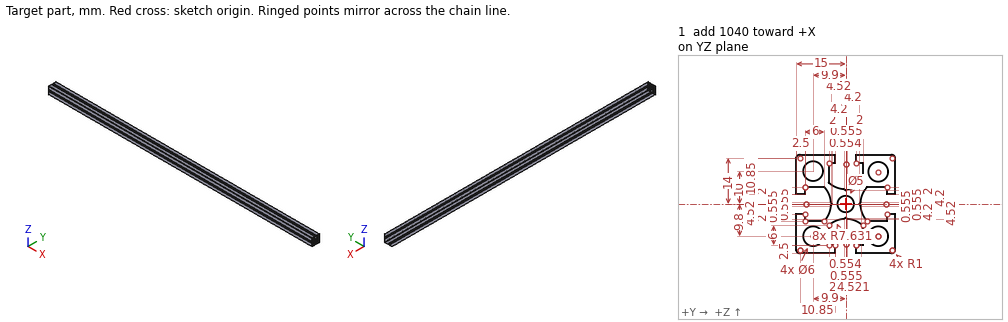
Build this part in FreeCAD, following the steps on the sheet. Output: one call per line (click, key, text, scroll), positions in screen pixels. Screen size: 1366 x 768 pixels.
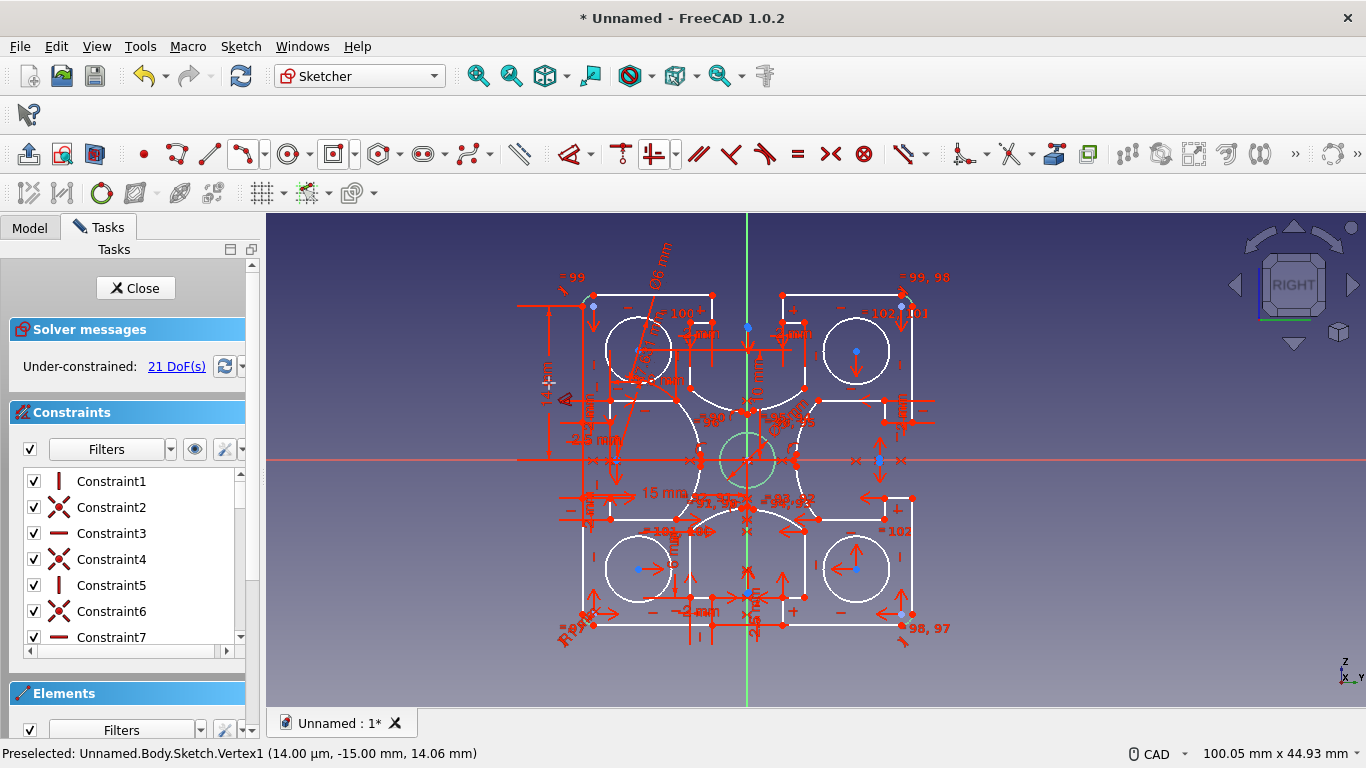
click(639, 350)
click(731, 292)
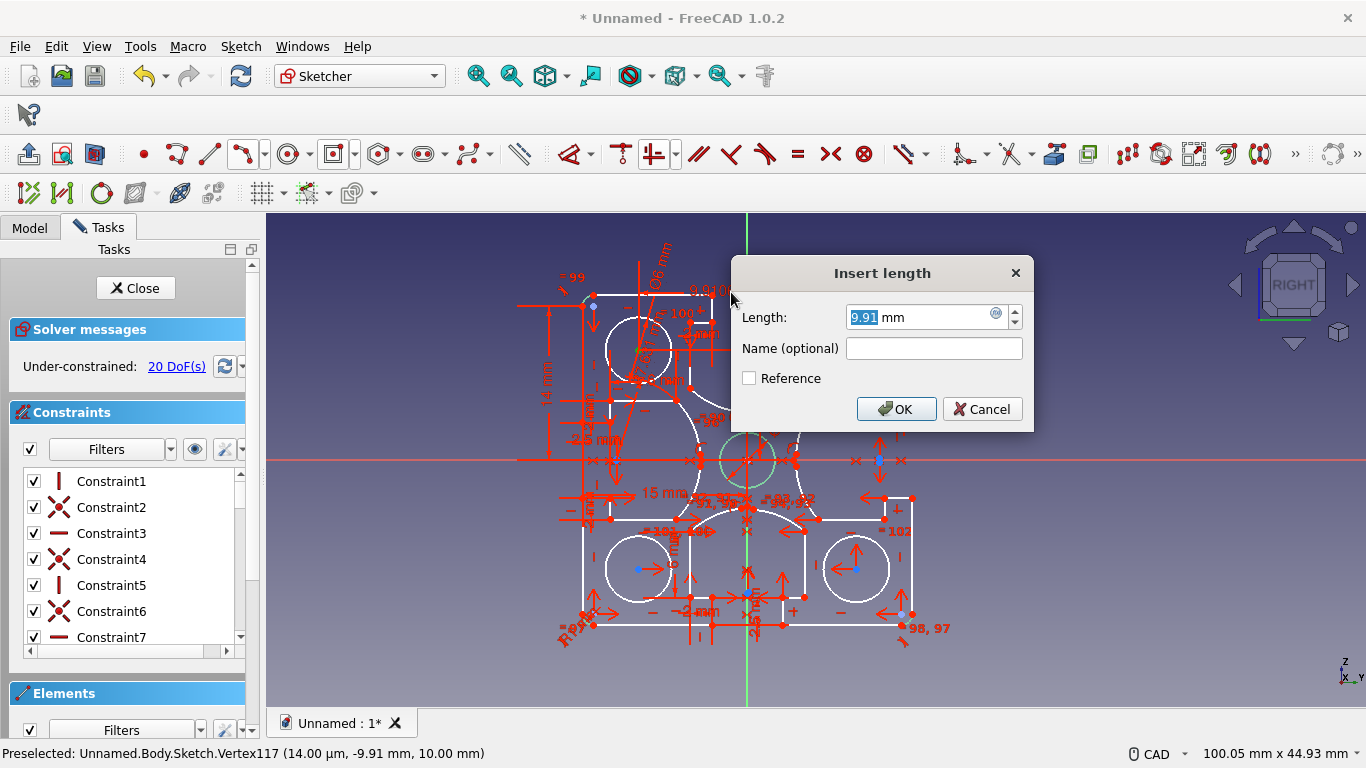
text(9.9)
key(Return)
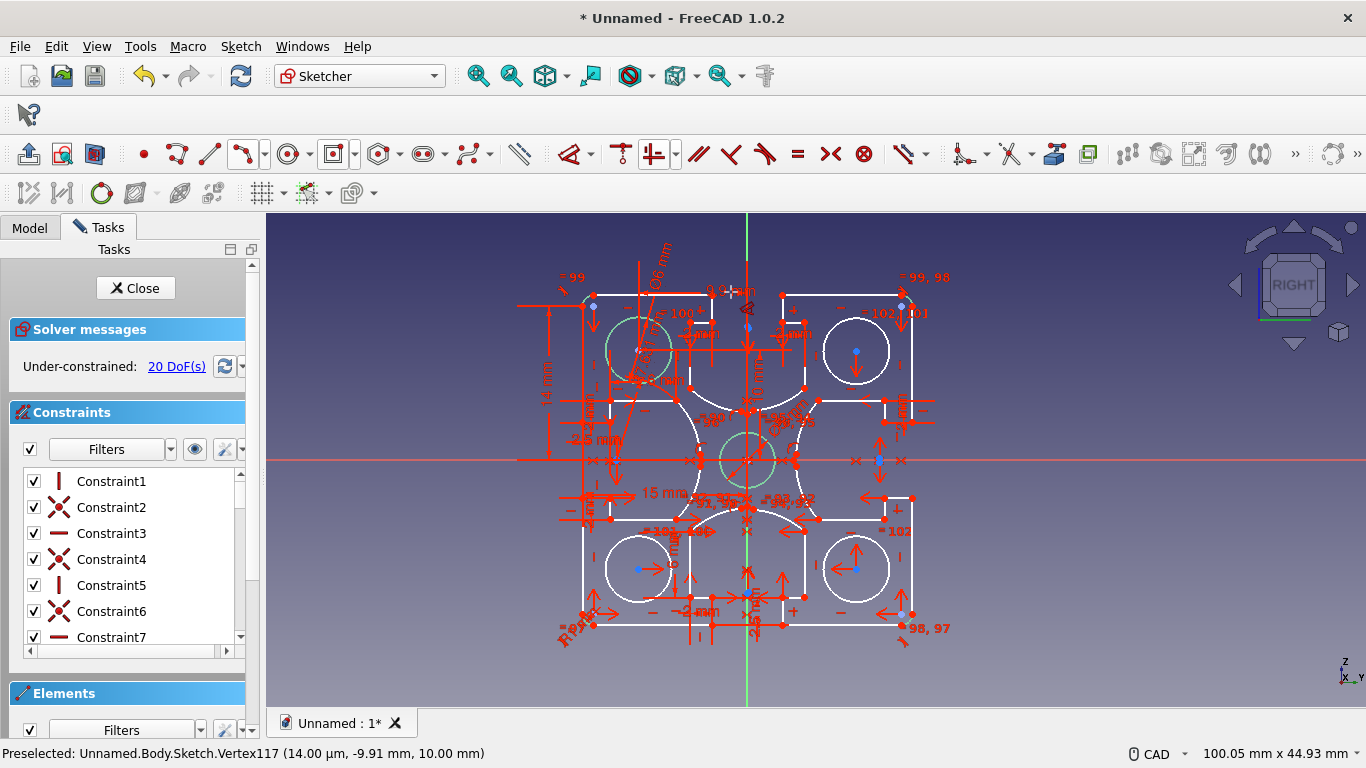
click(639, 569)
click(668, 426)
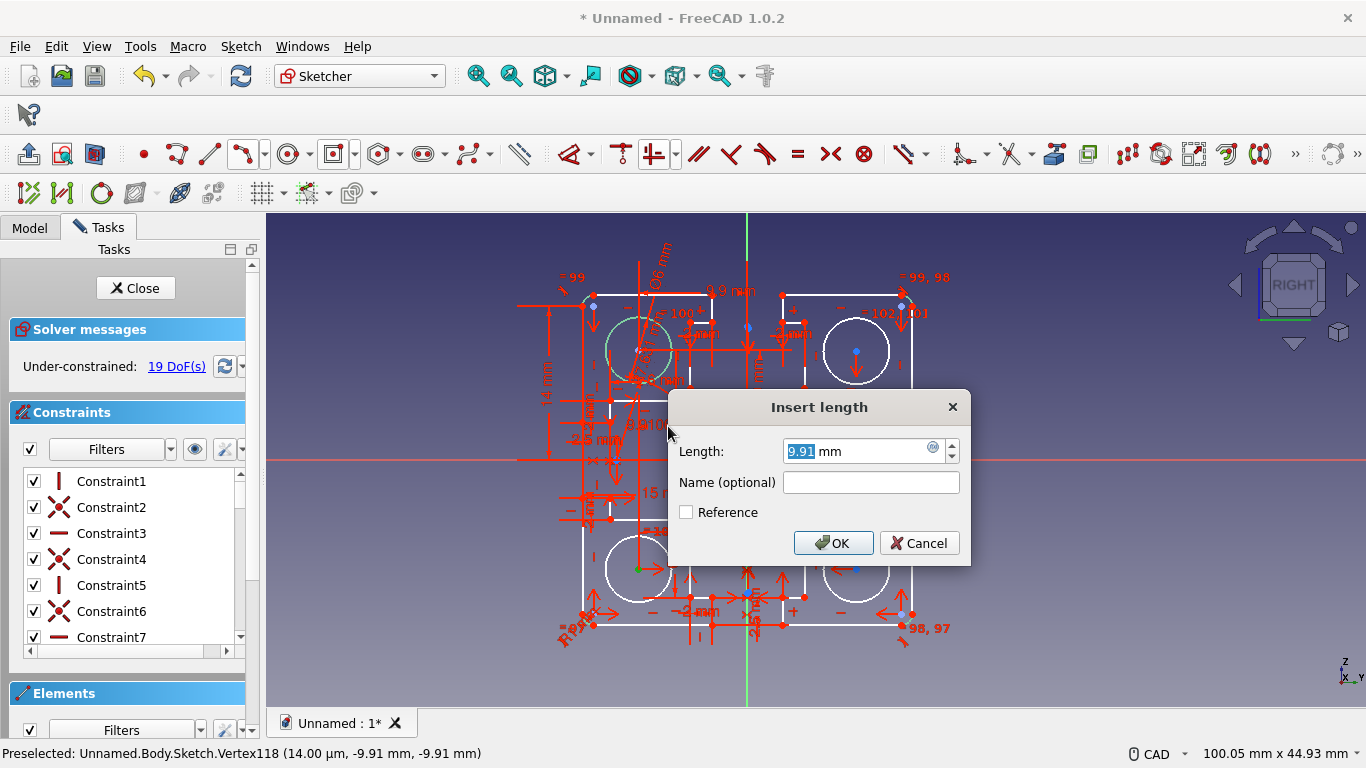
text(9.9)
key(Return)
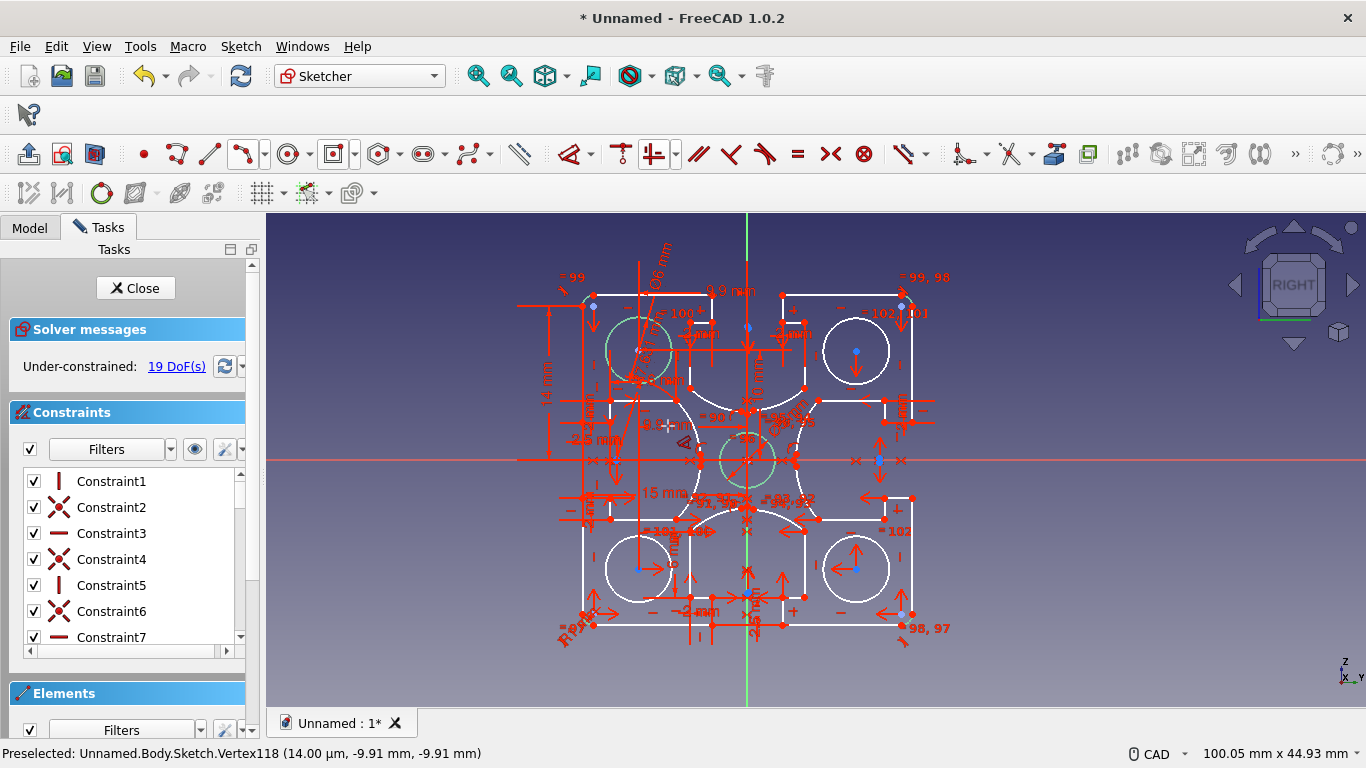
click(639, 569)
click(781, 490)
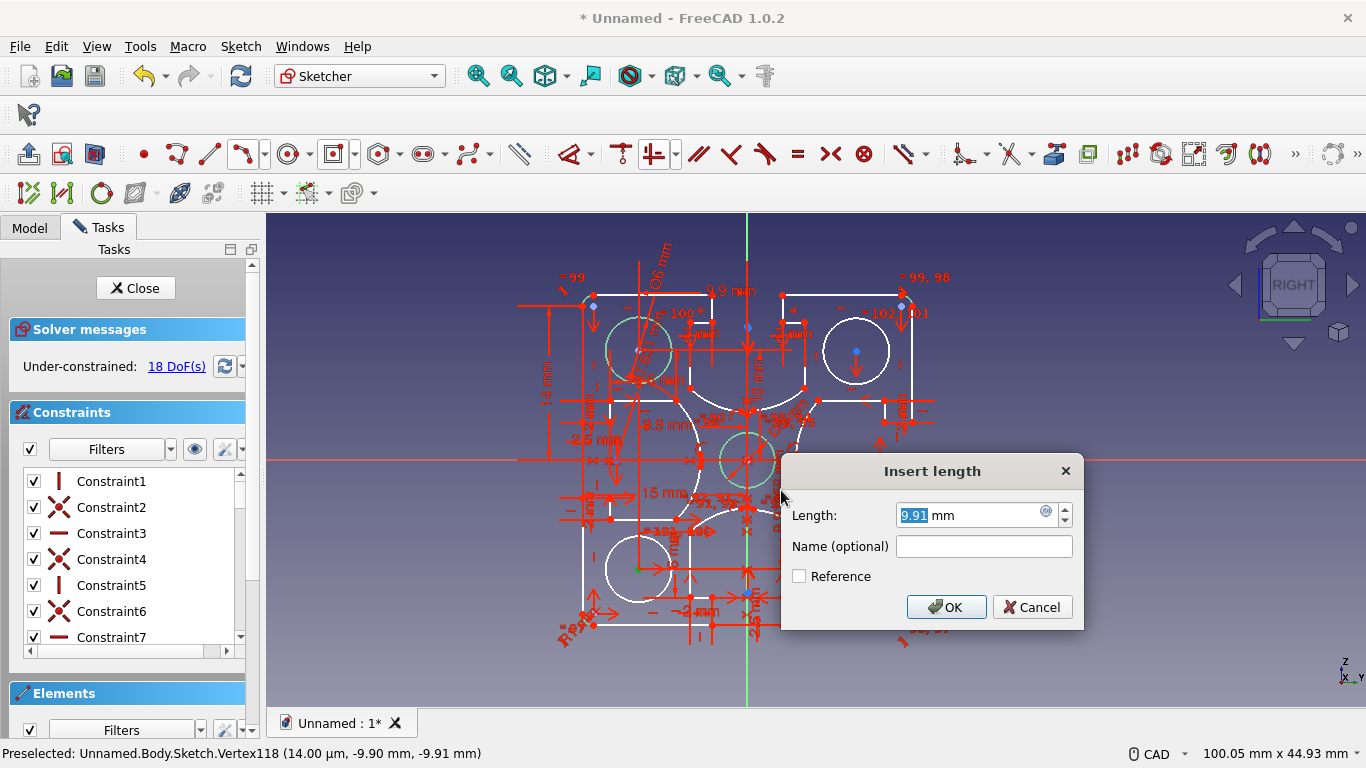
text(9.8)
key(Return)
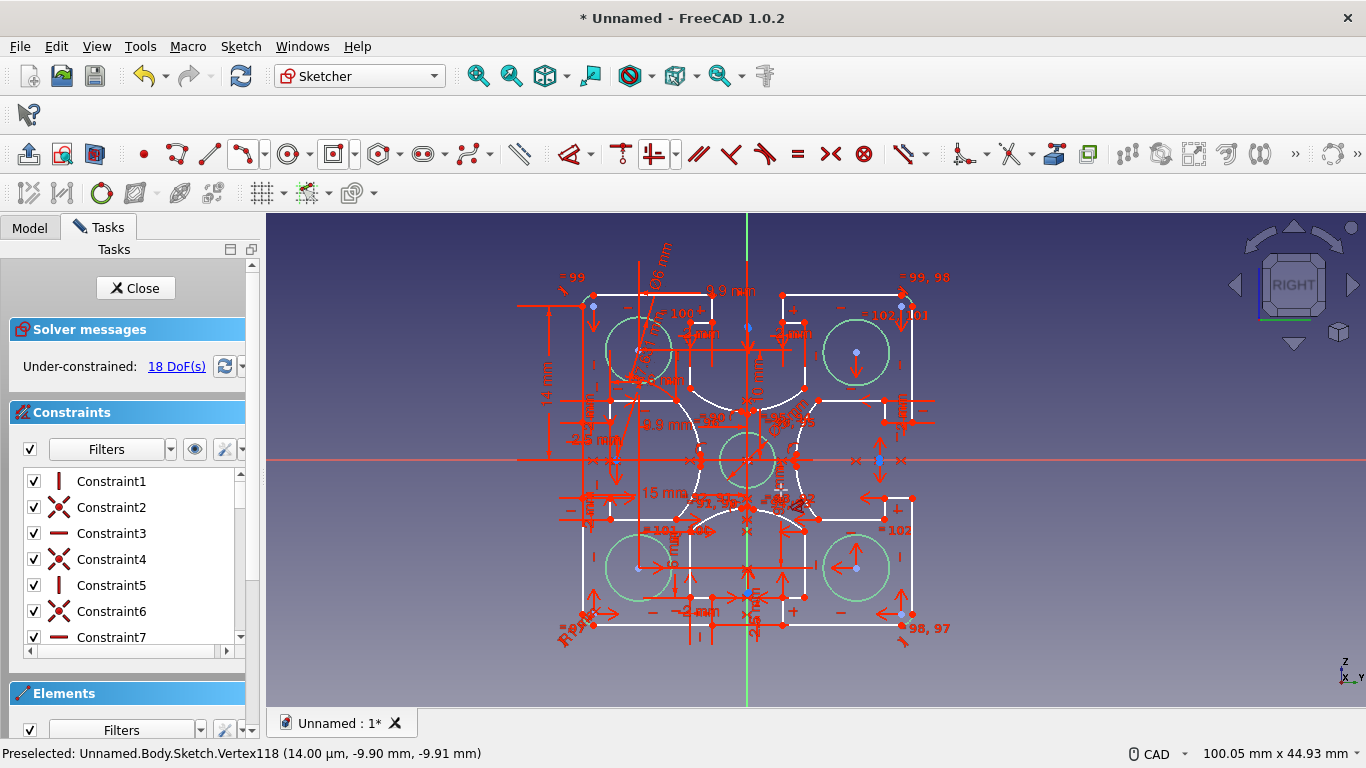
scroll(701, 460, up, 4)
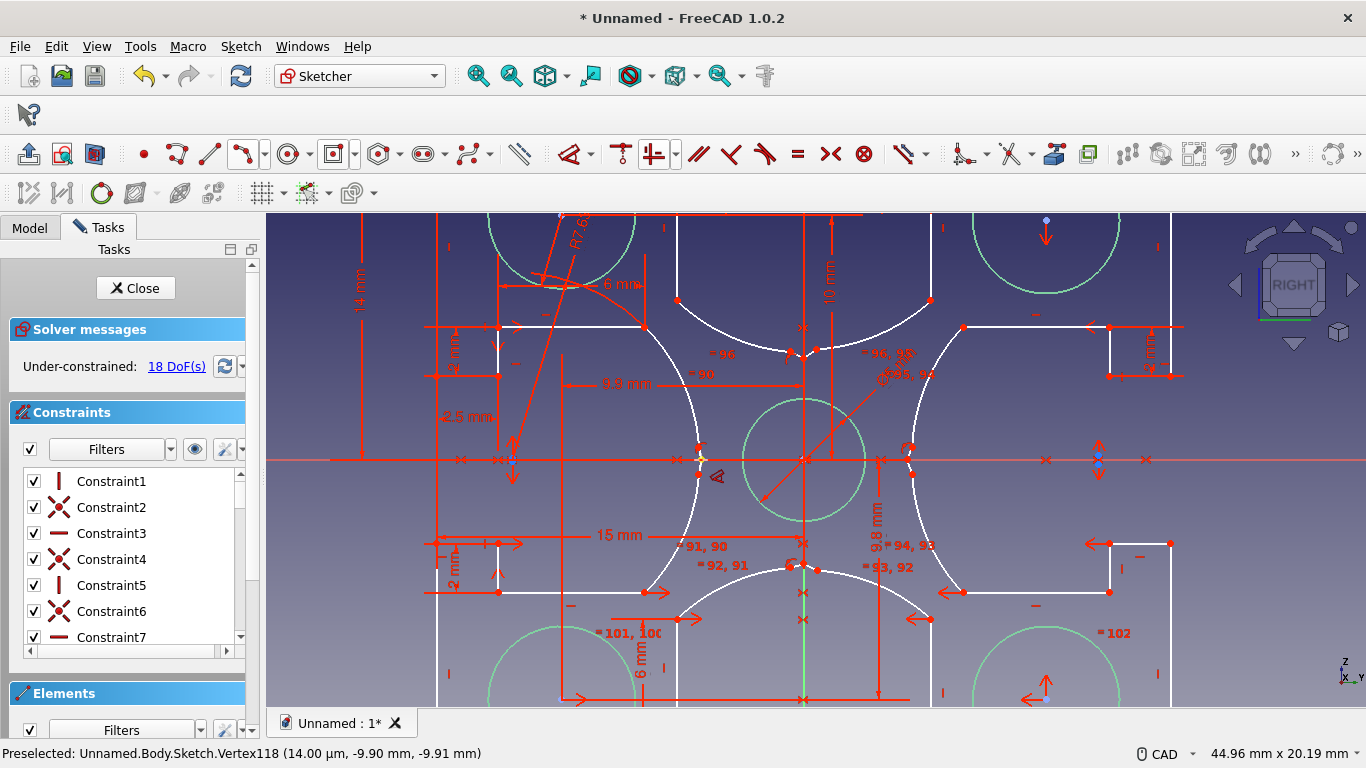
click(701, 460)
click(729, 494)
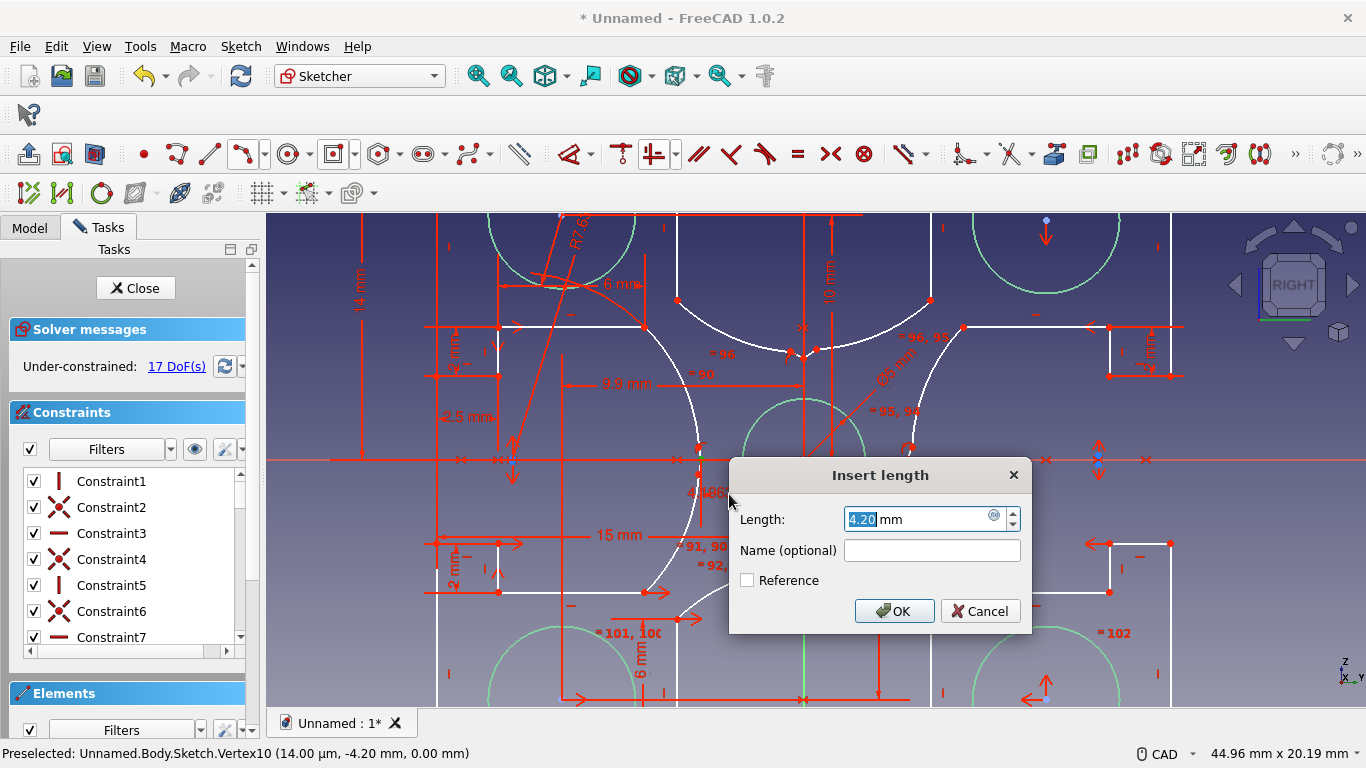
text(4.2)
key(Return)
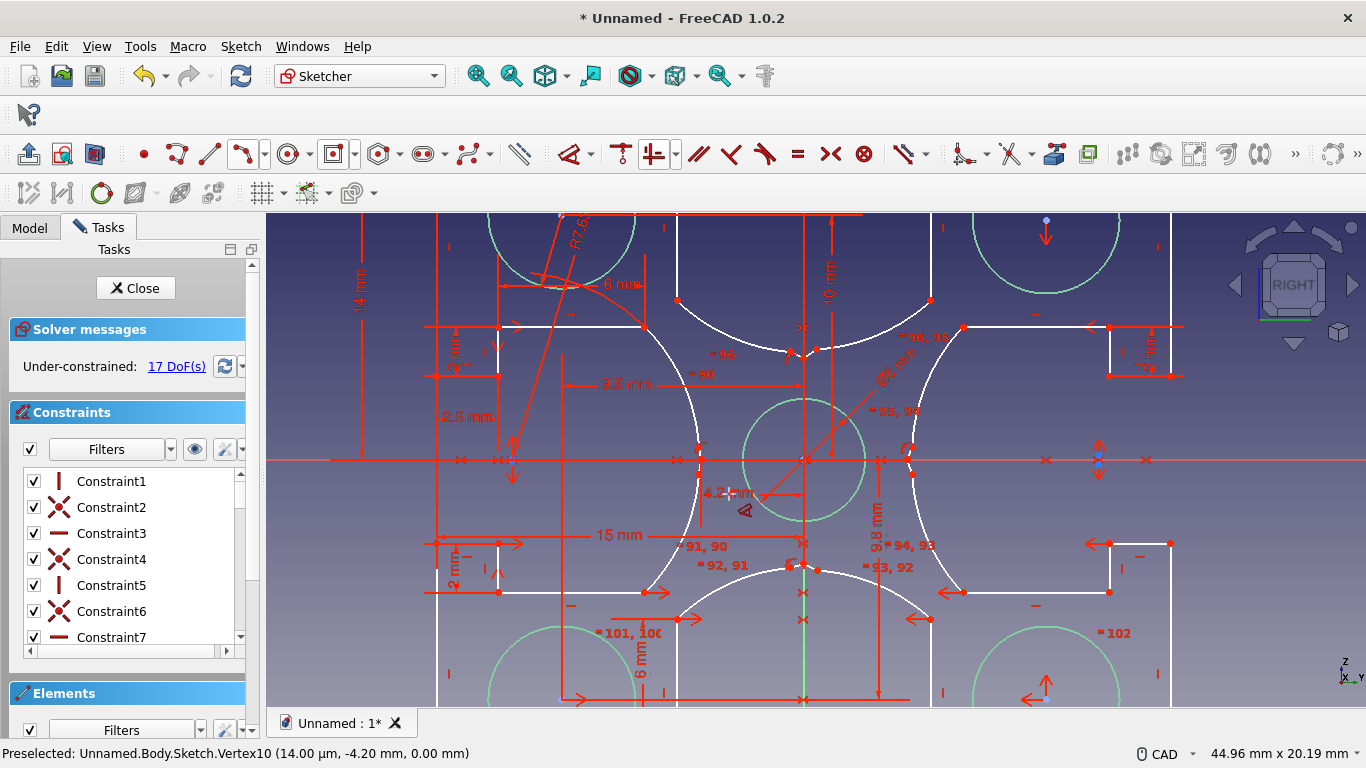
click(804, 564)
click(838, 488)